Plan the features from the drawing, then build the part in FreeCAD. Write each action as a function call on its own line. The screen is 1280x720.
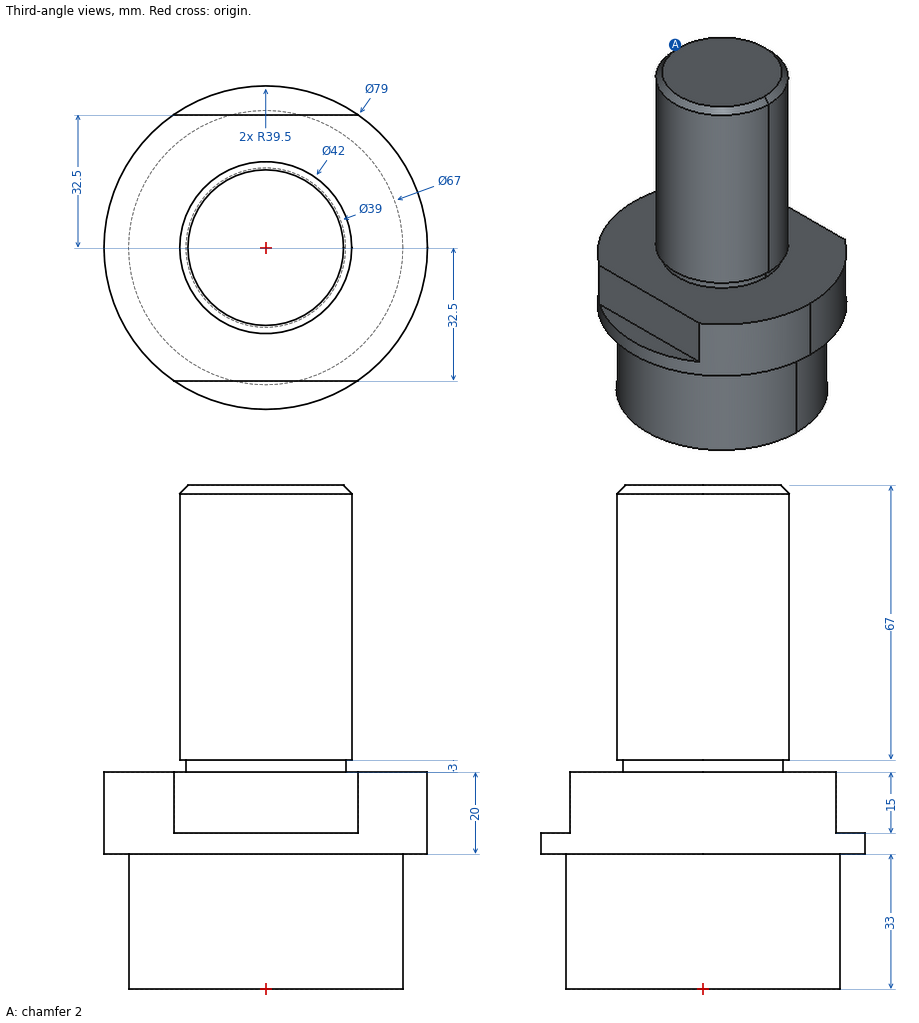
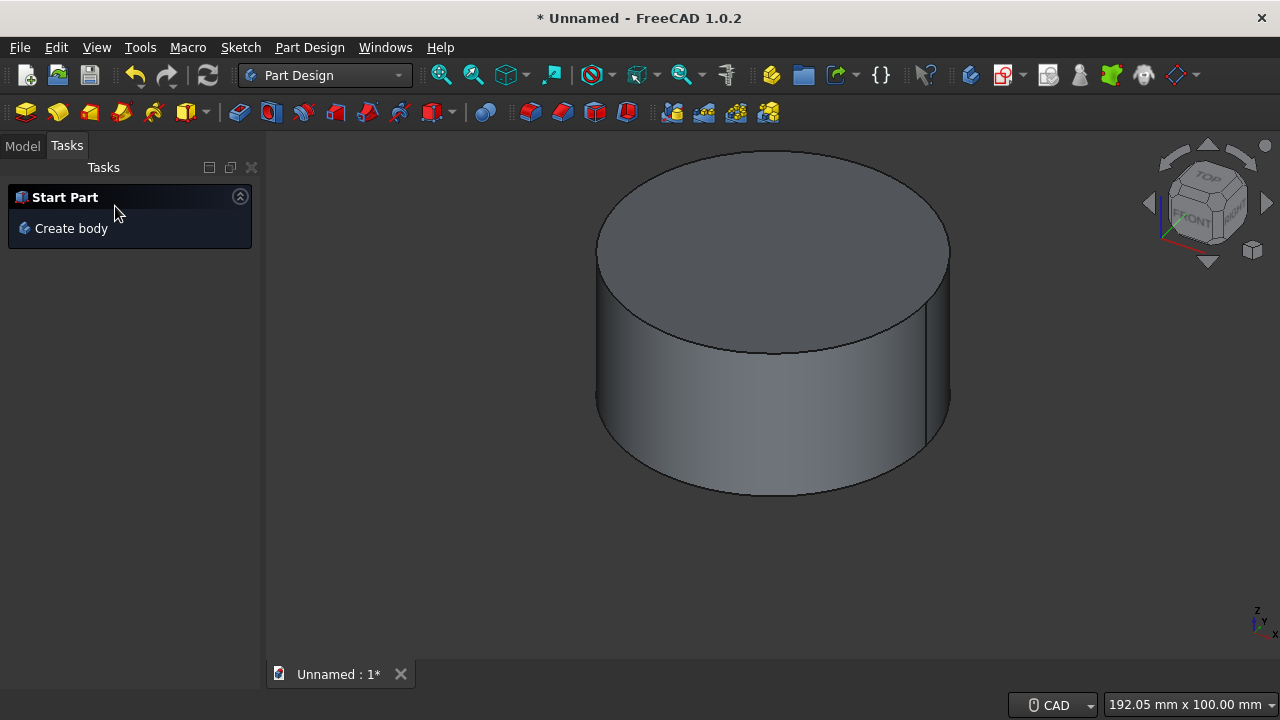
click(442, 76)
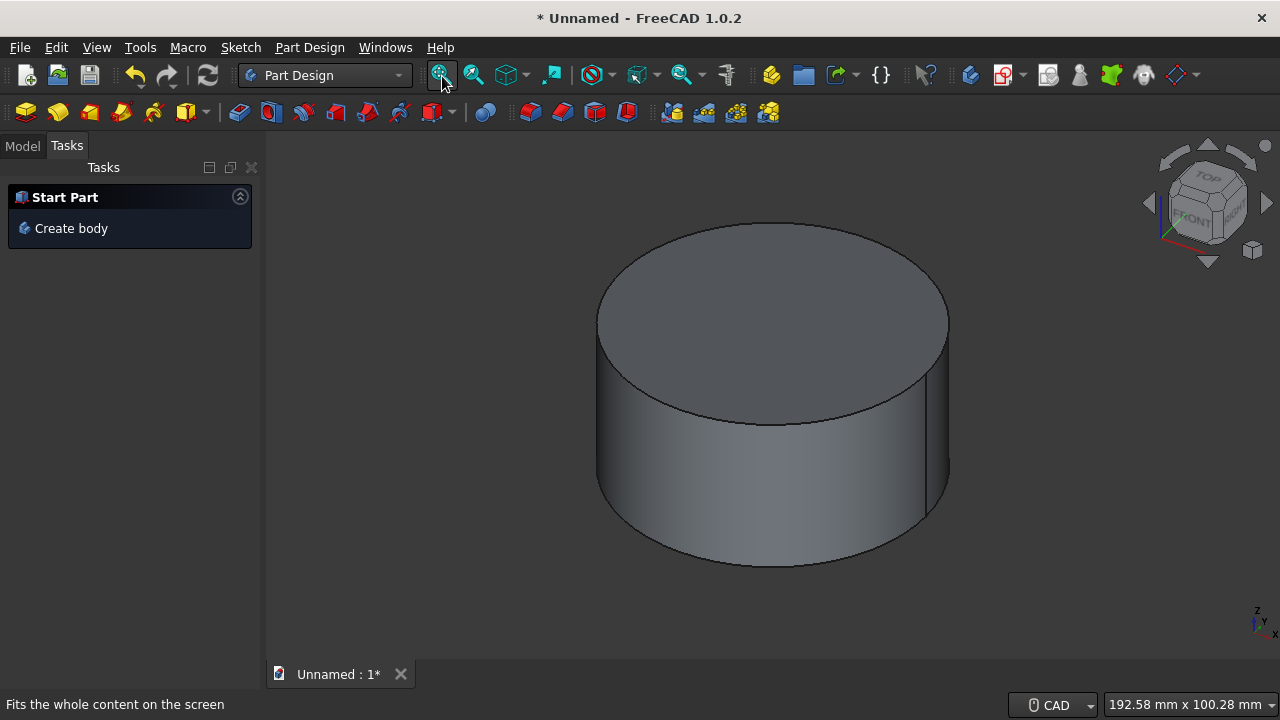
click(773, 323)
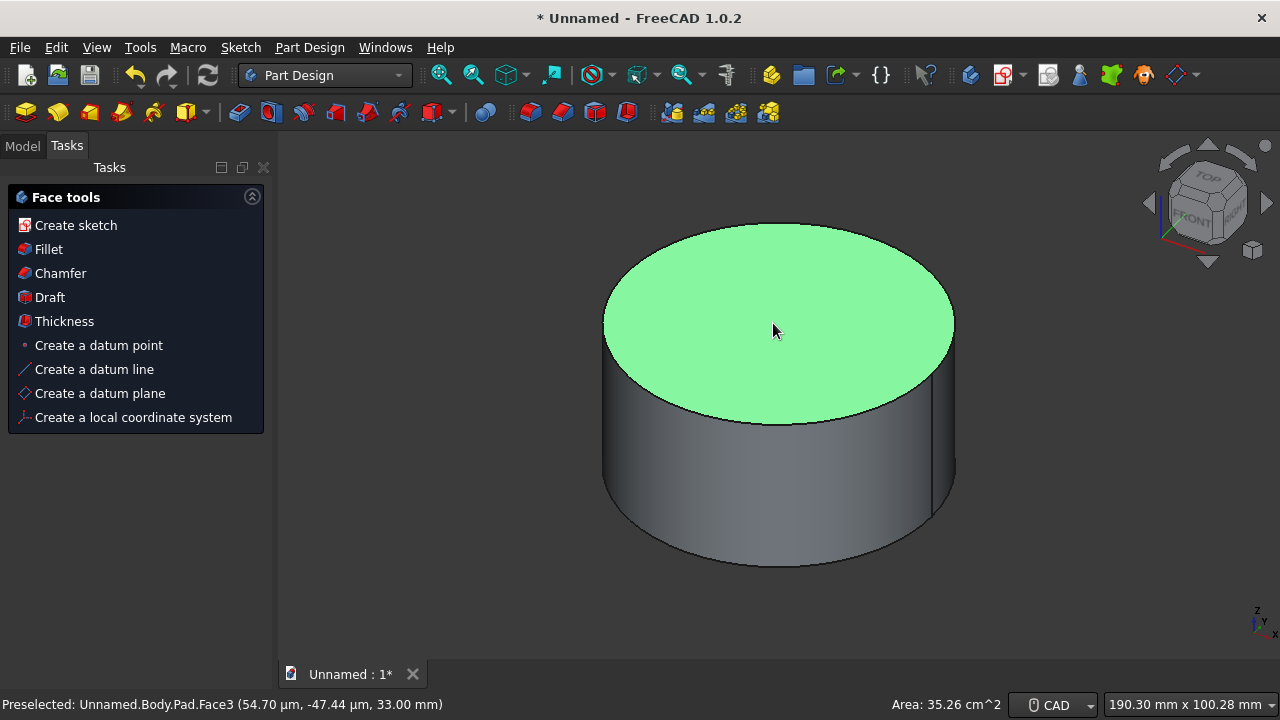
click(1004, 76)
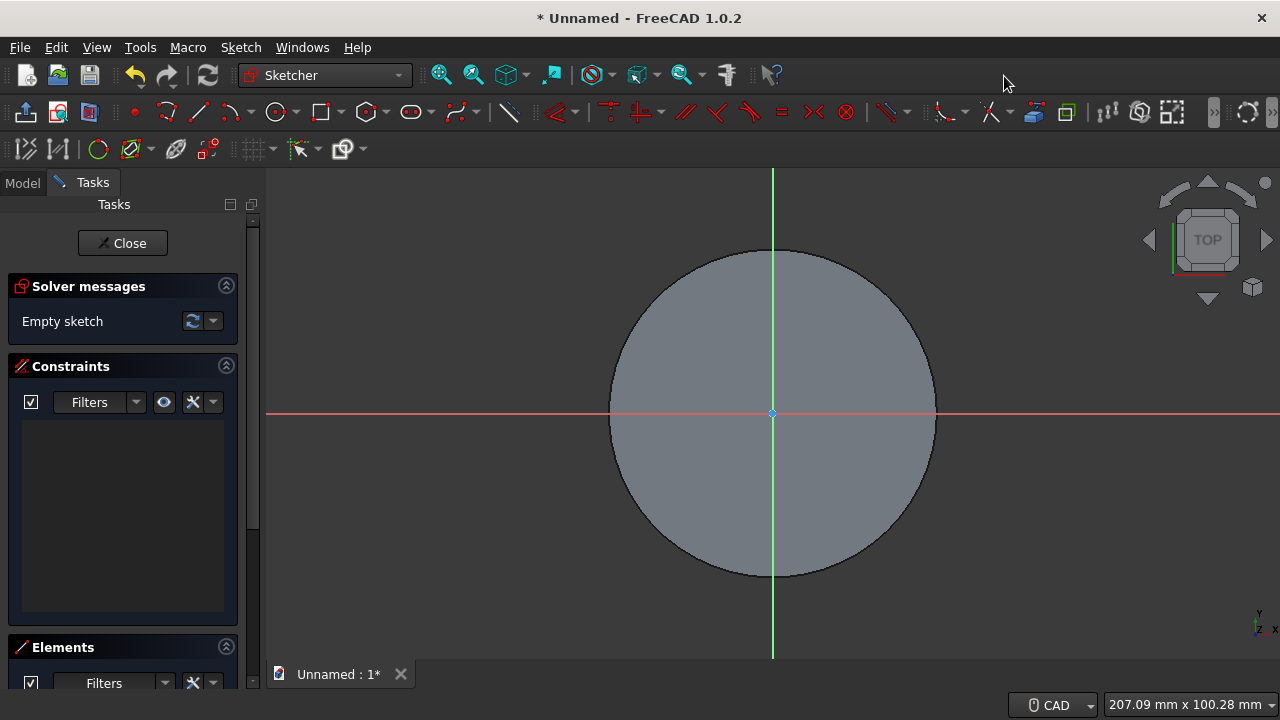
scroll(396, 413, down, 1)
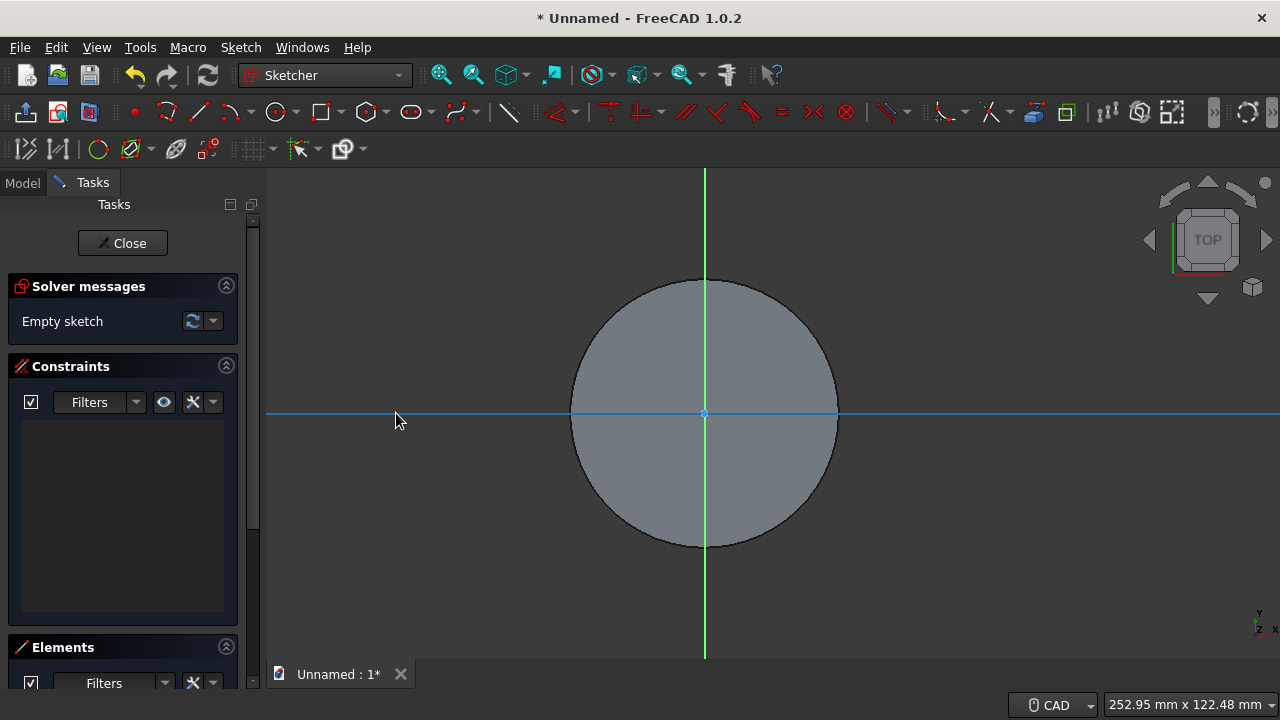
click(276, 112)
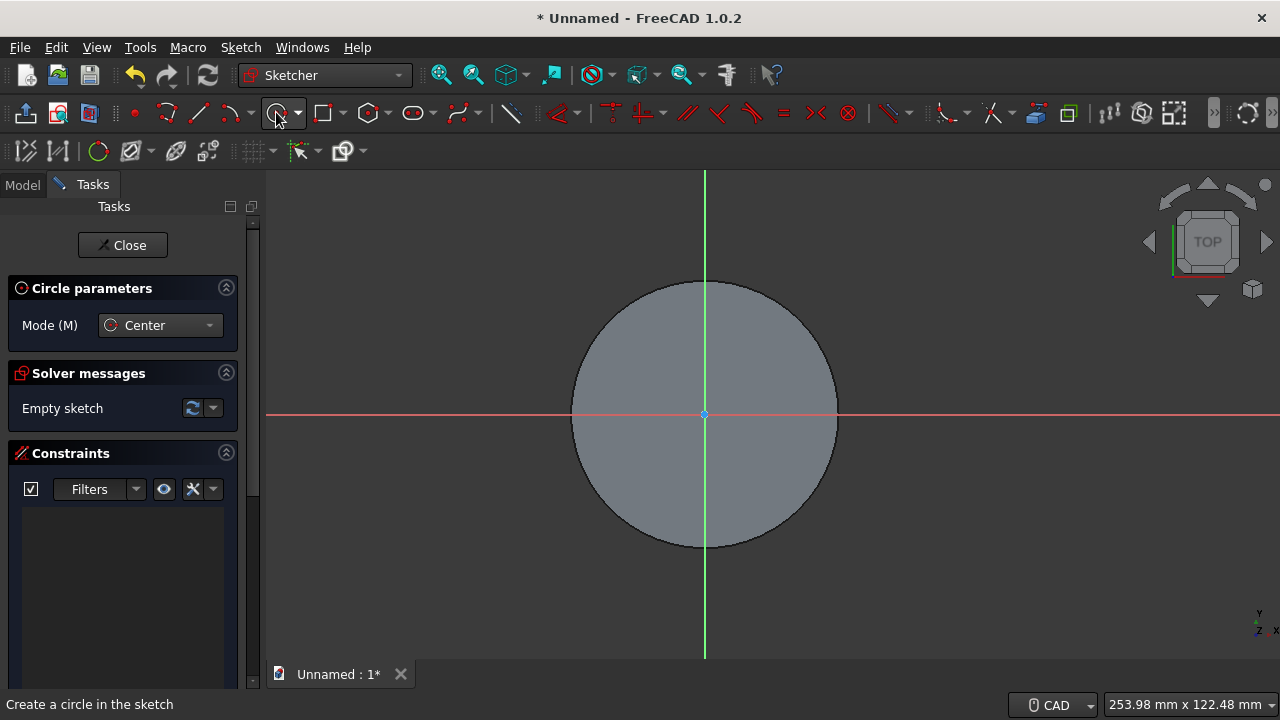
click(705, 414)
move(816, 303)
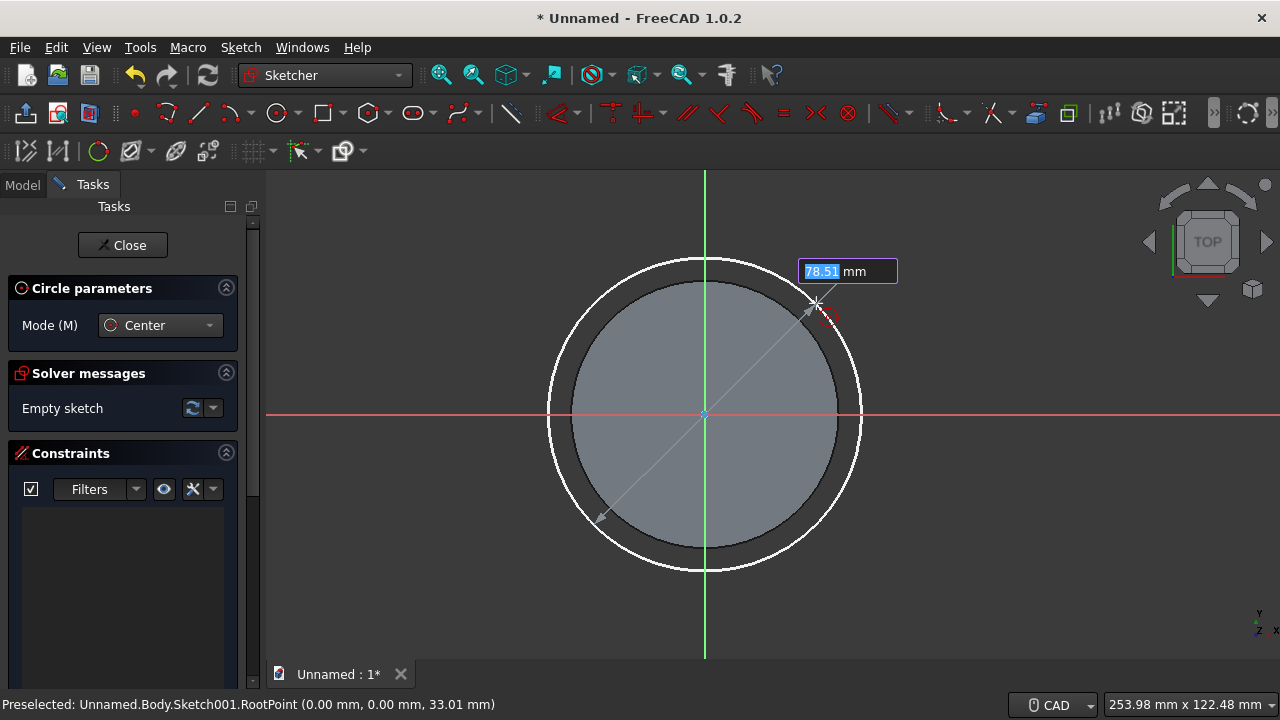
text(79)
key(Return)
key(Escape)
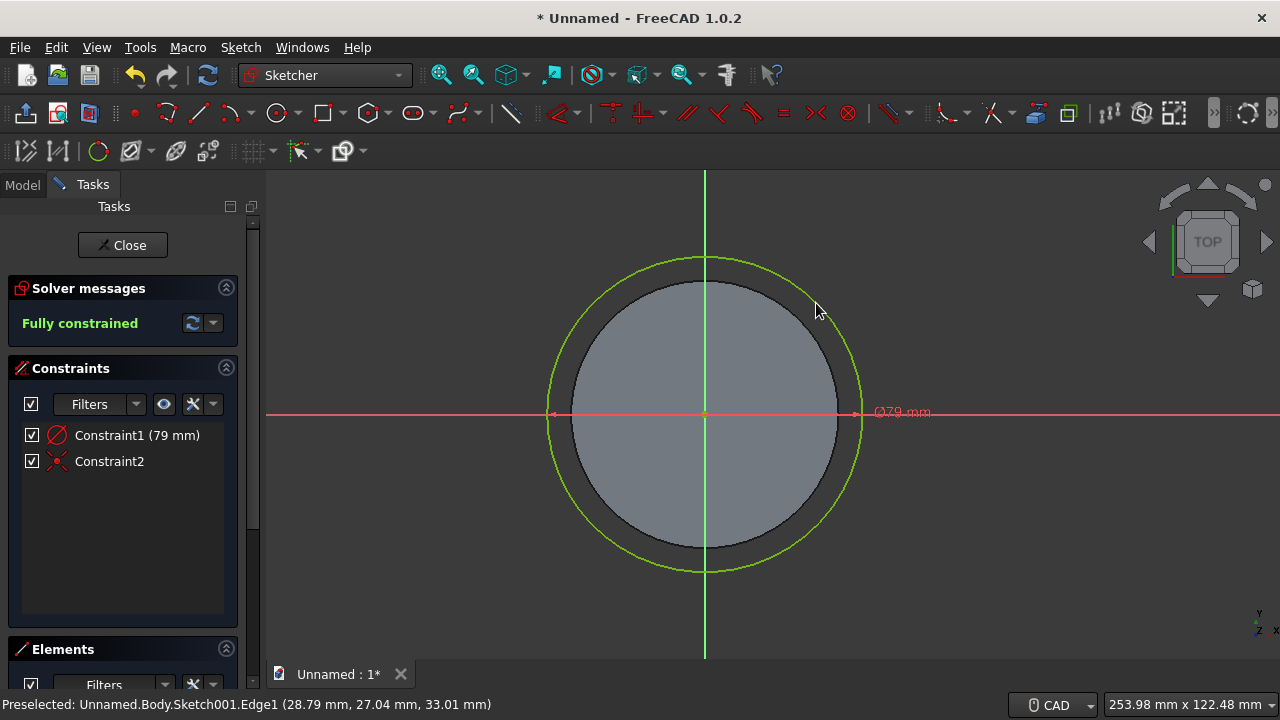
click(123, 245)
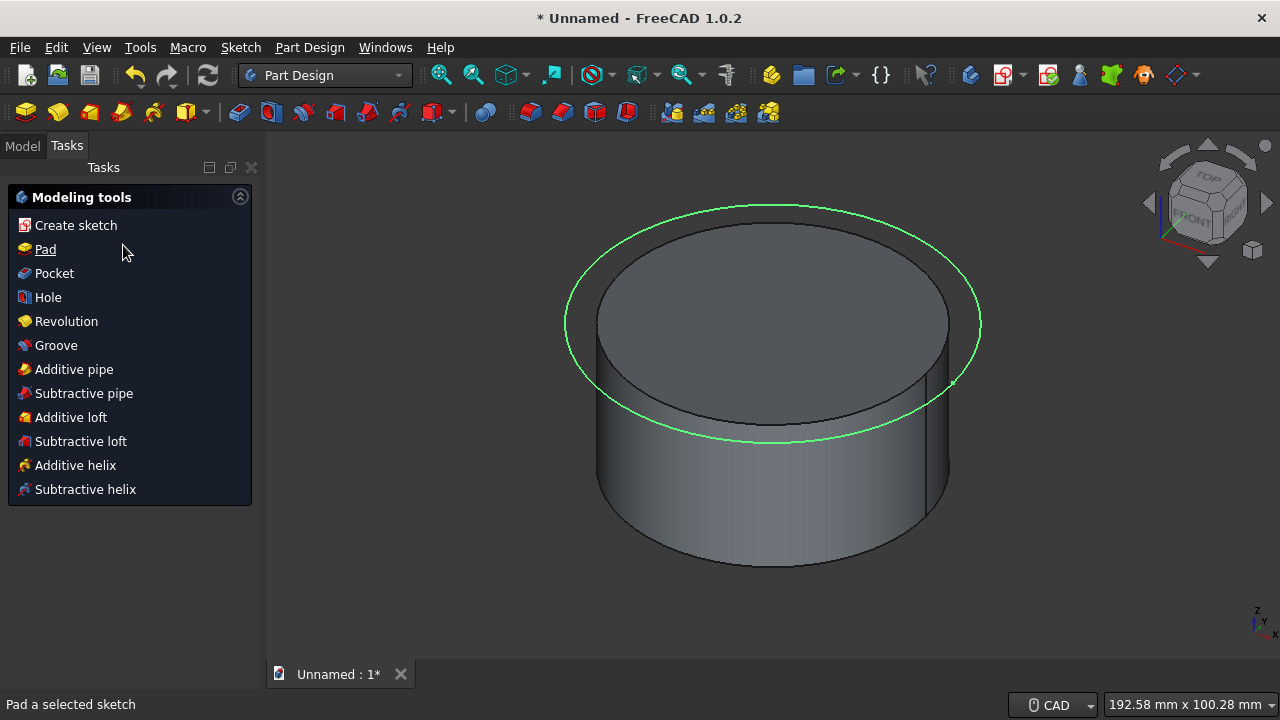
click(26, 112)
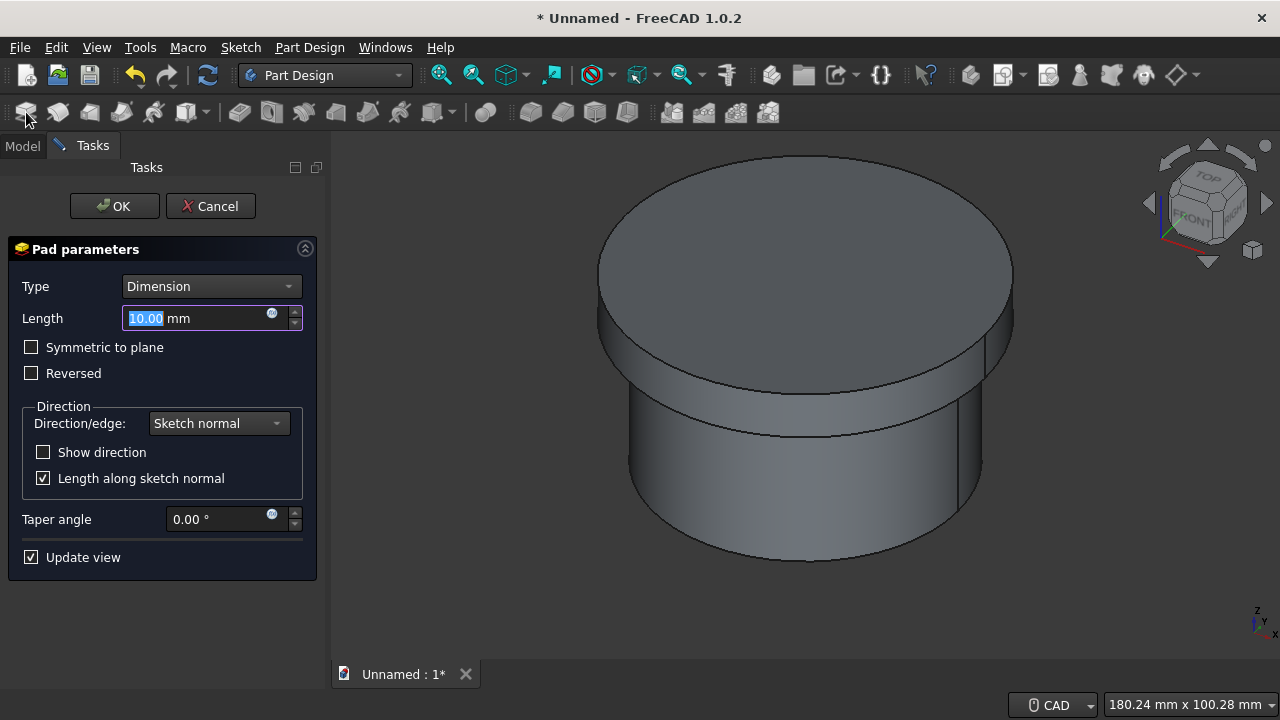
text(20)
key(Tab)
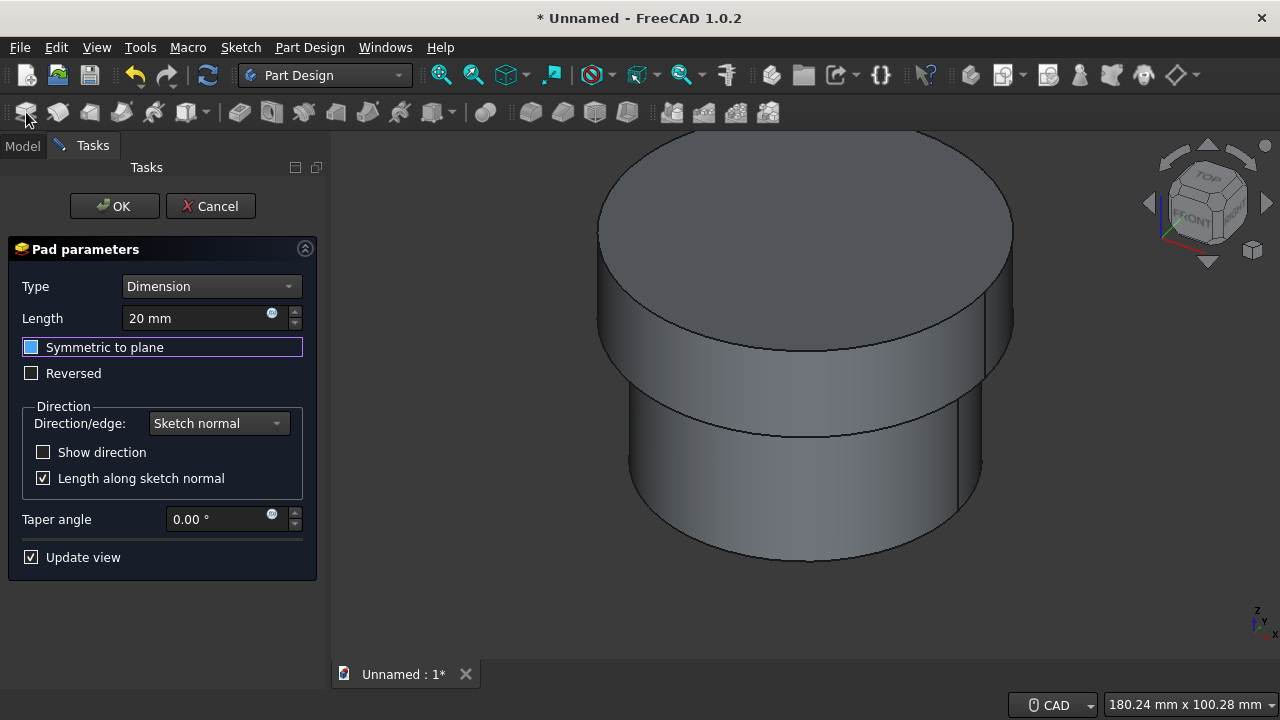
click(115, 206)